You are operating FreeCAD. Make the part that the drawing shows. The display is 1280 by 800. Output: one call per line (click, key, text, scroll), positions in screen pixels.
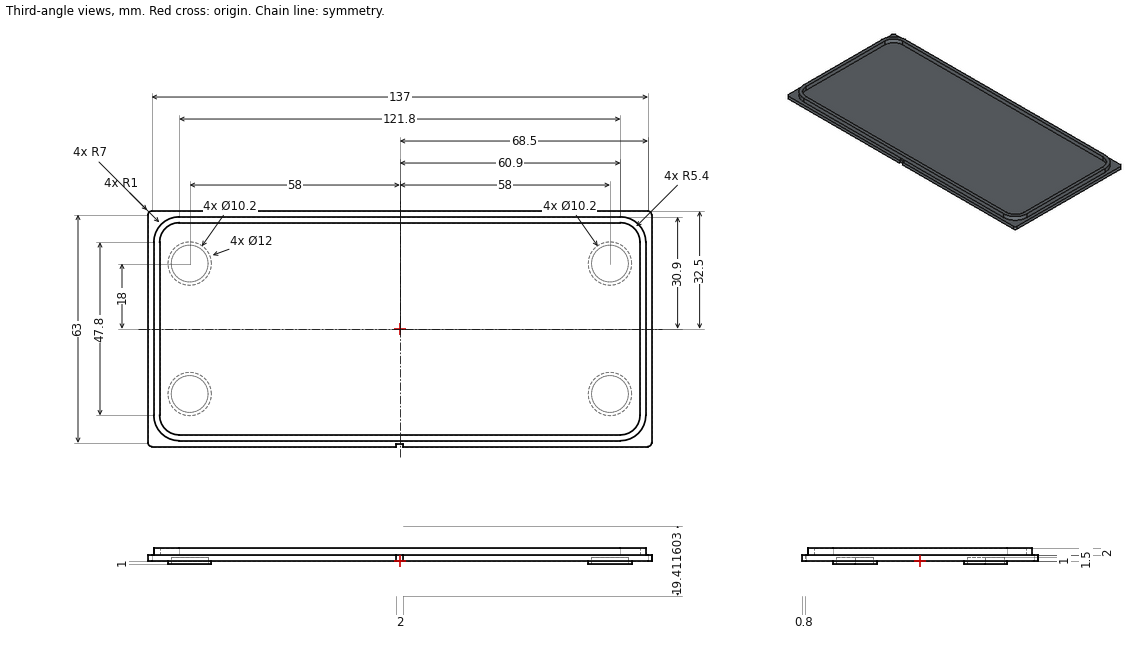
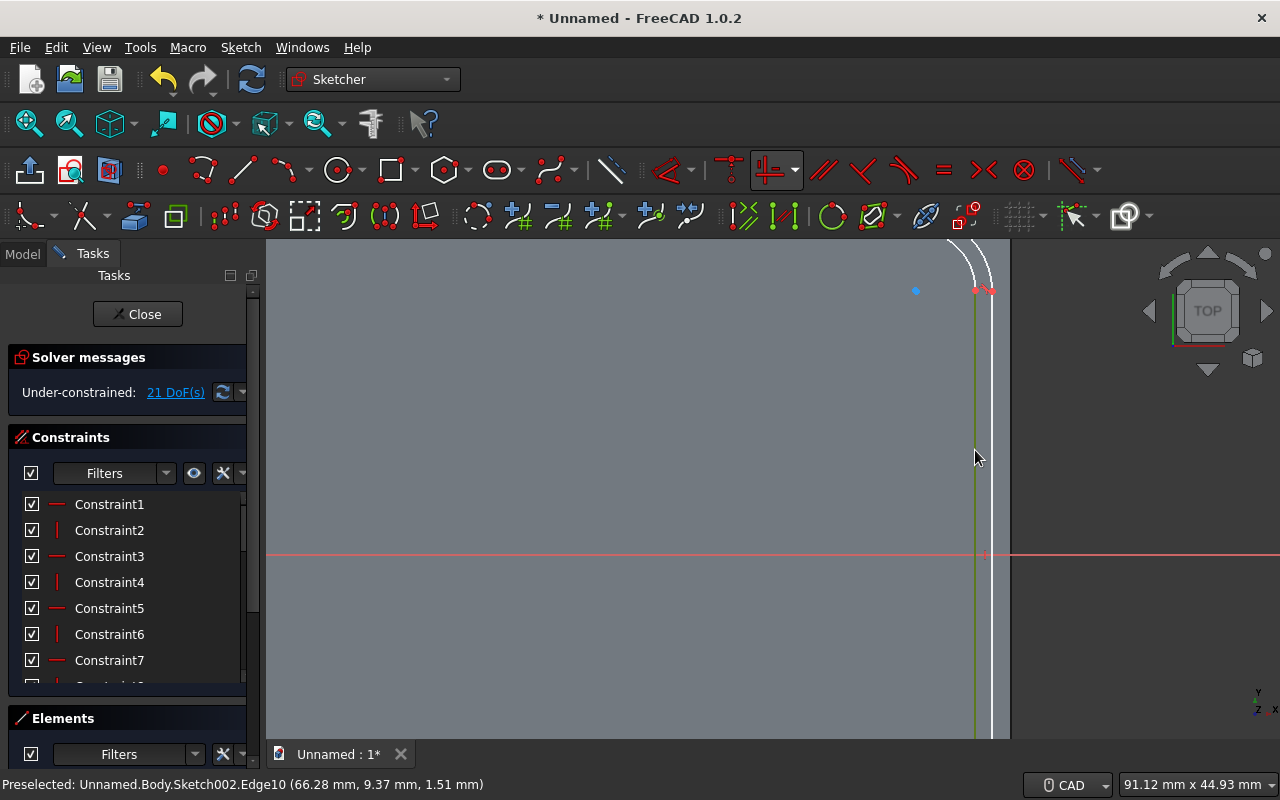
scroll(976, 450, down, 5)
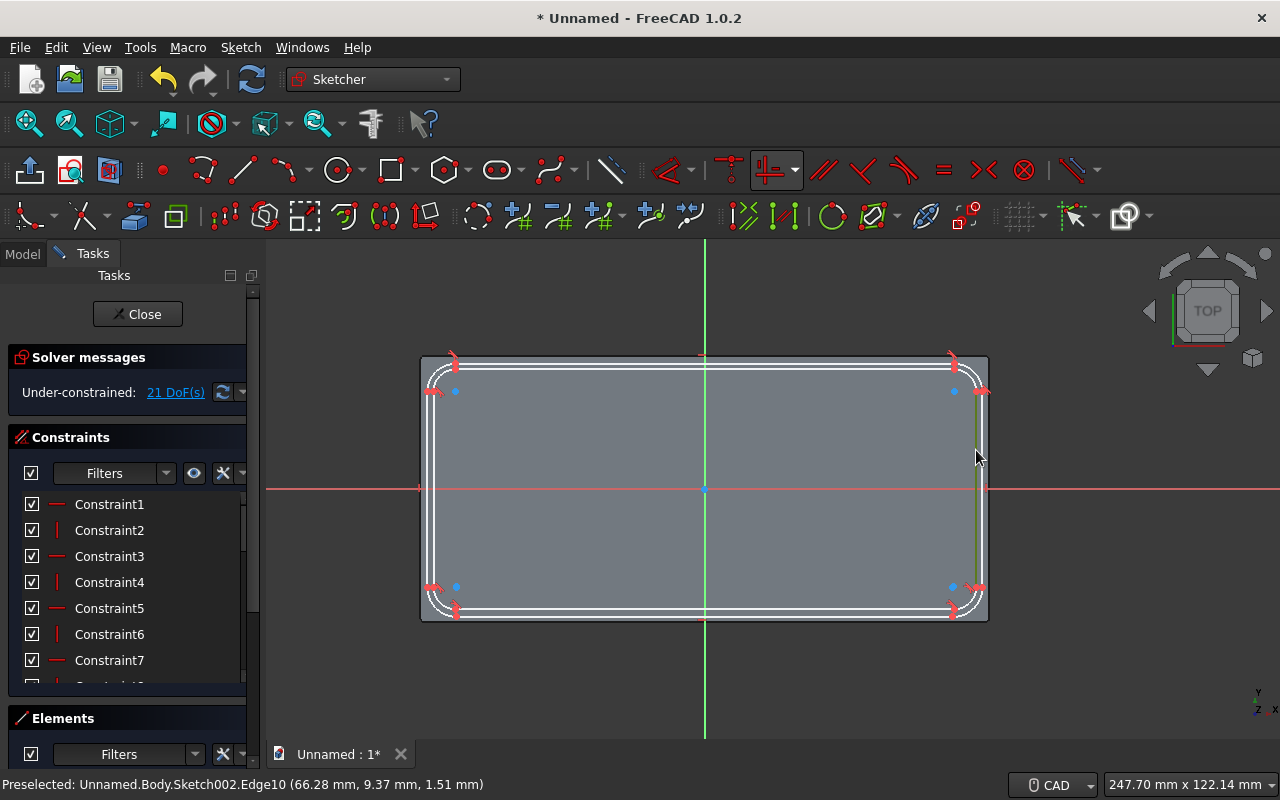
scroll(964, 607, up, 4)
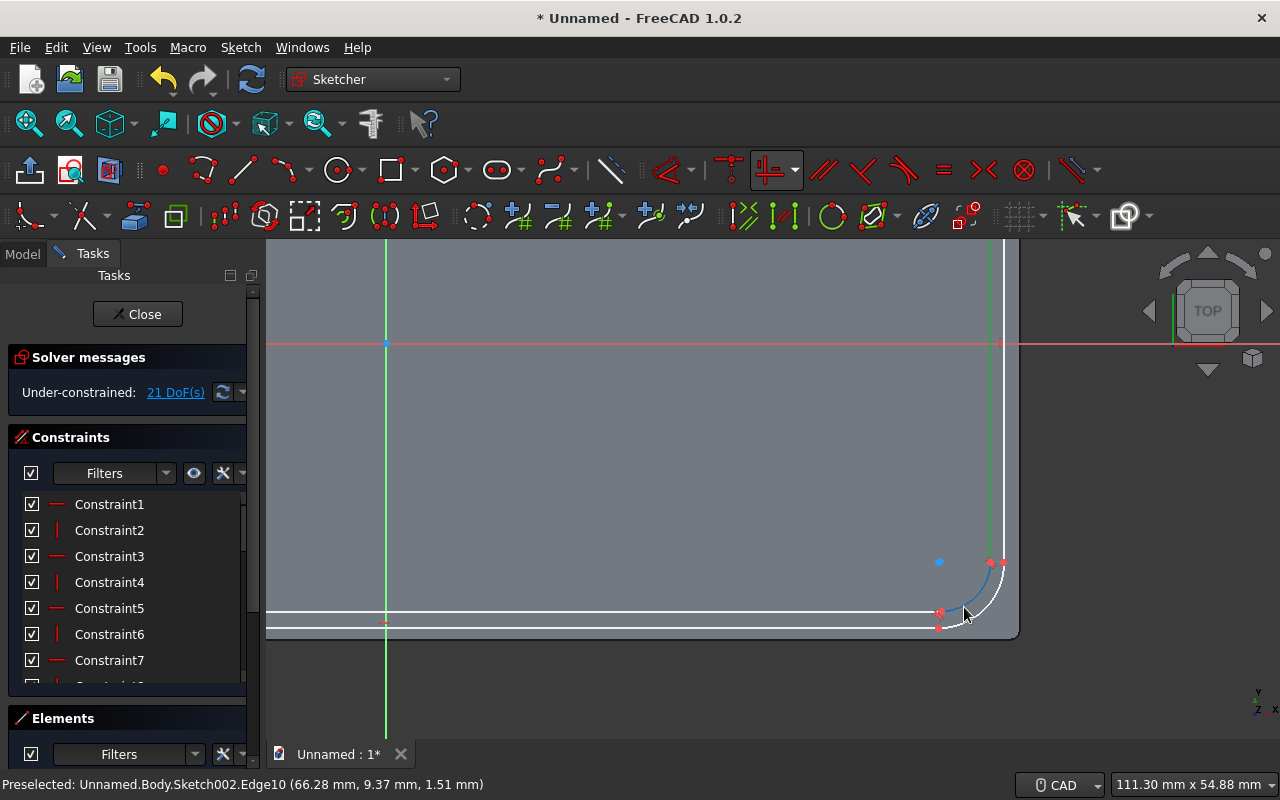
click(963, 606)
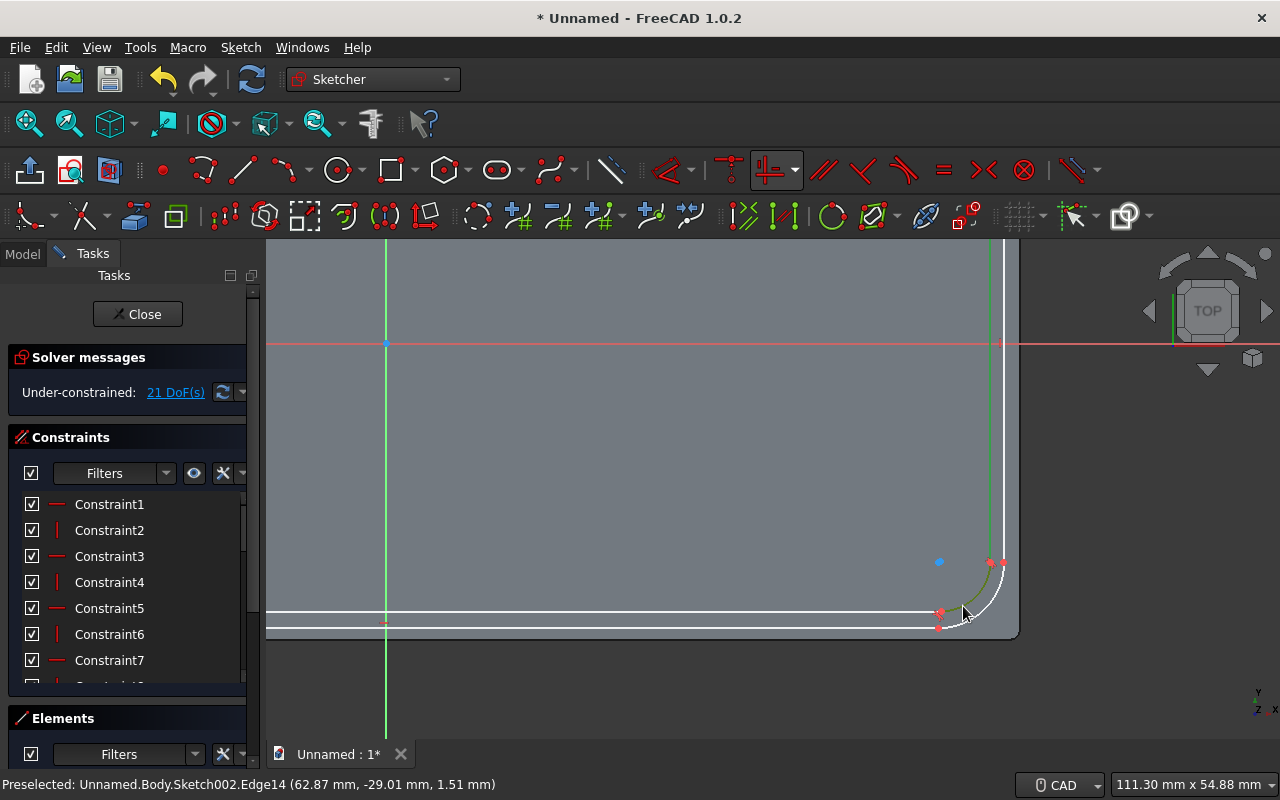
click(904, 170)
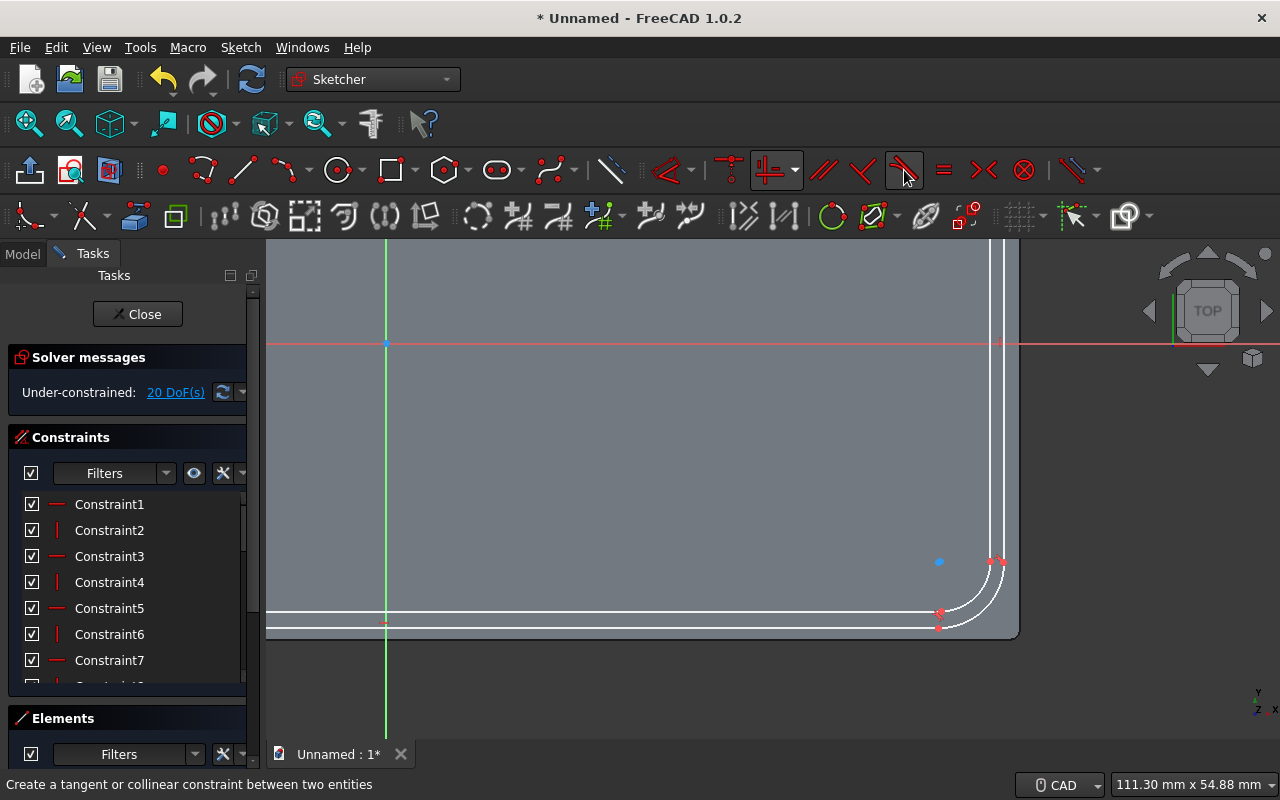
click(608, 612)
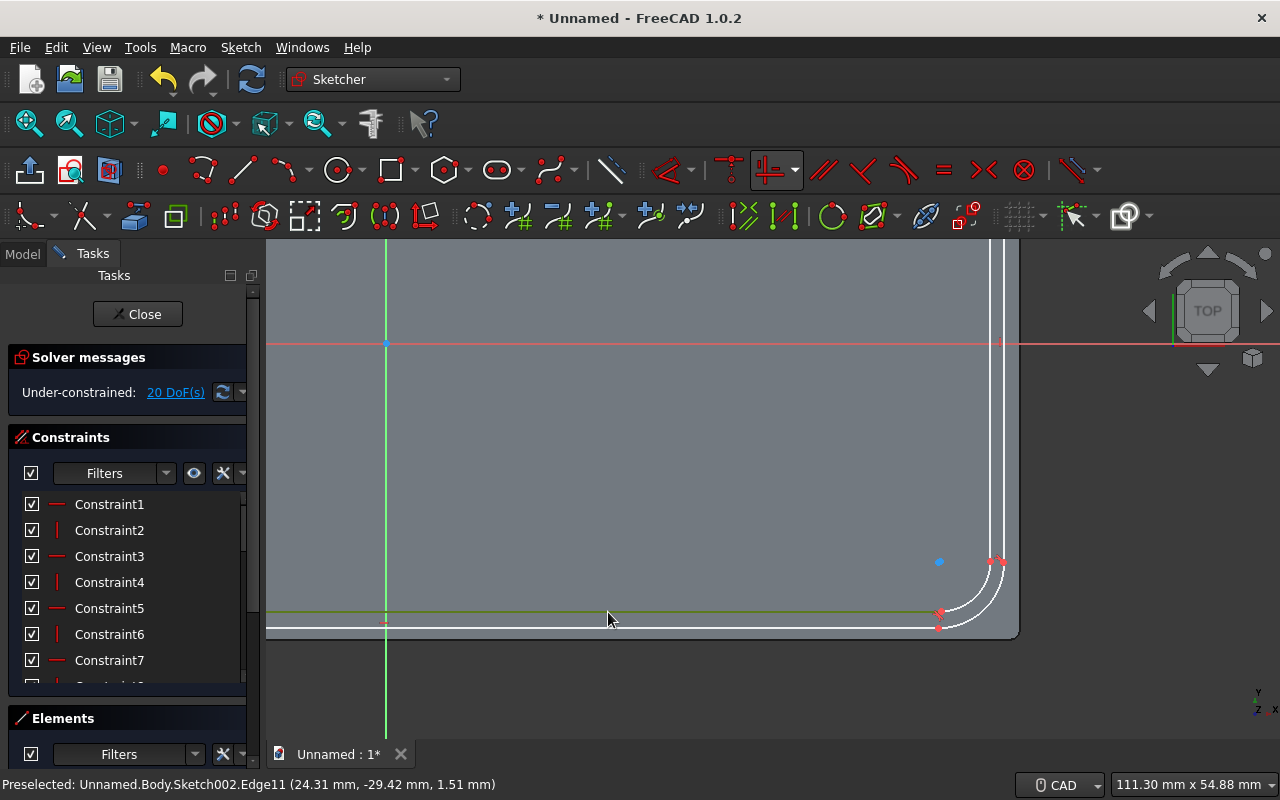
click(964, 606)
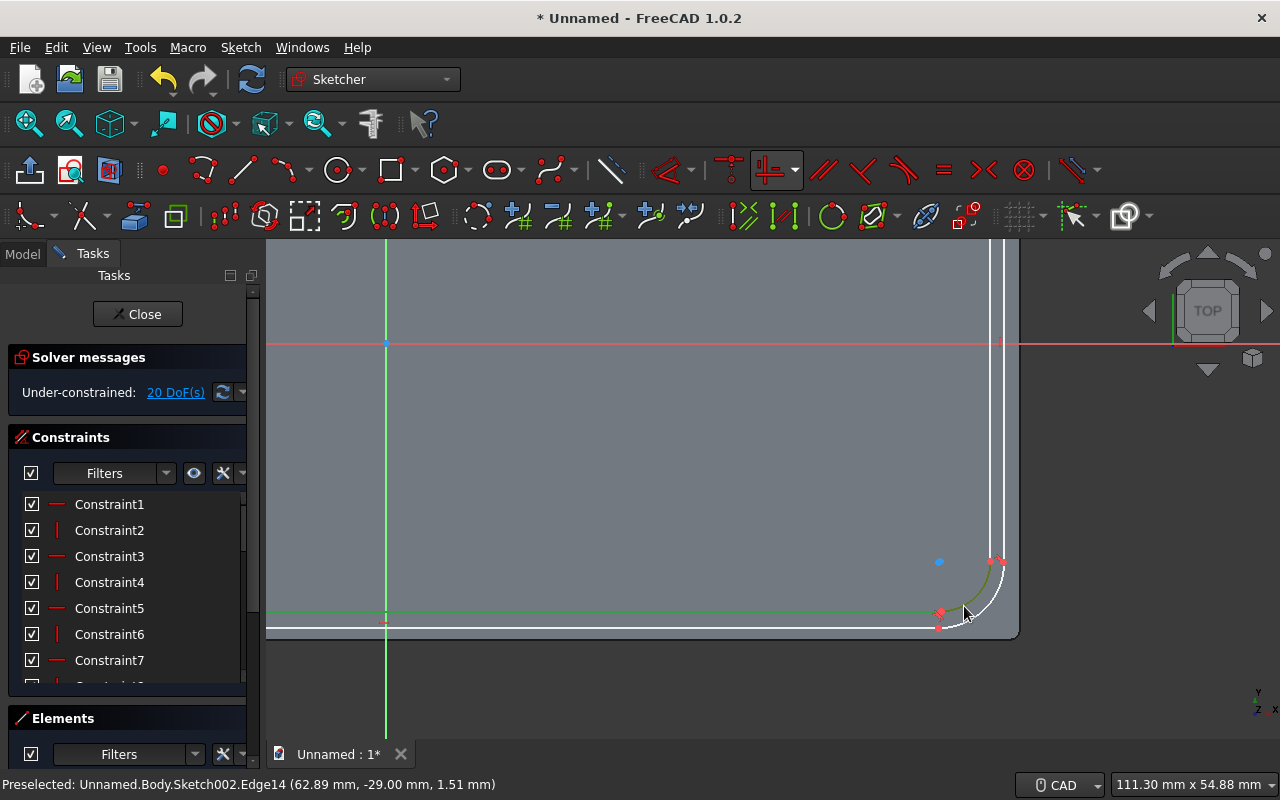
click(904, 170)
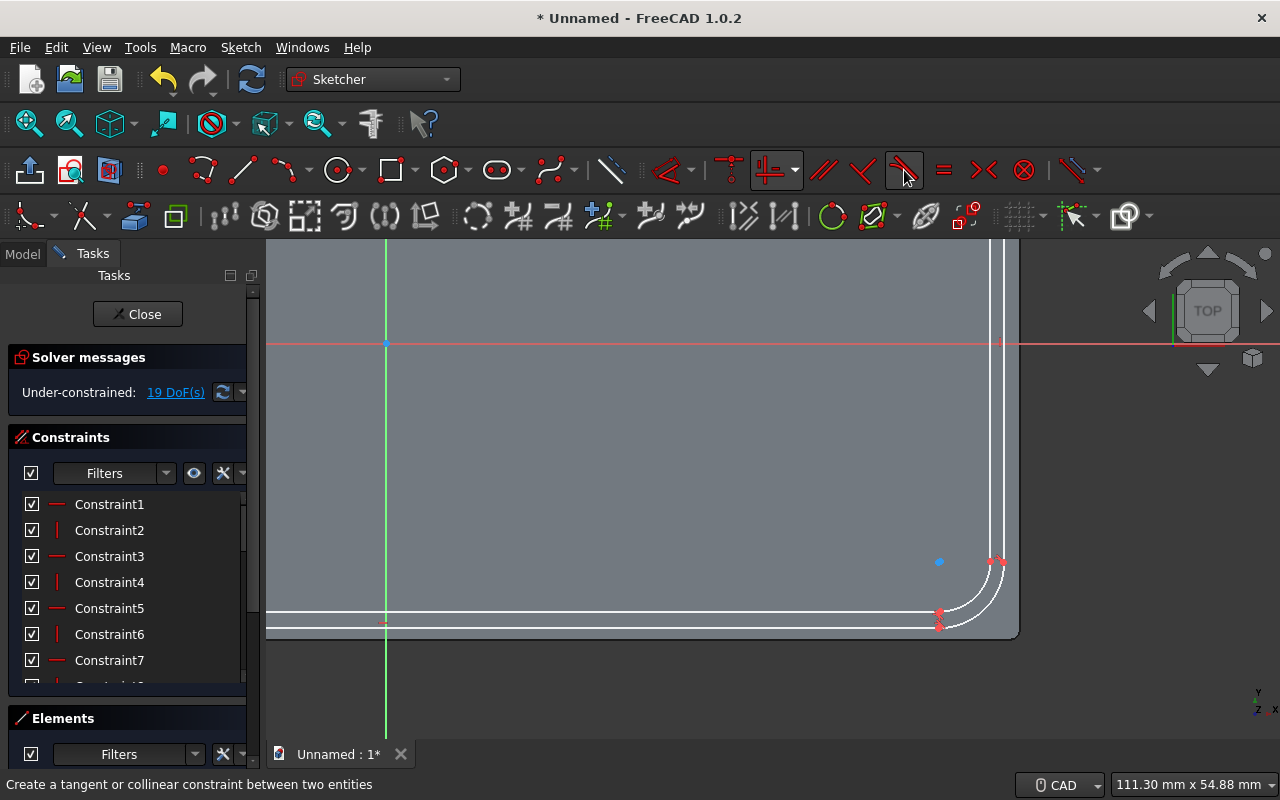
click(608, 612)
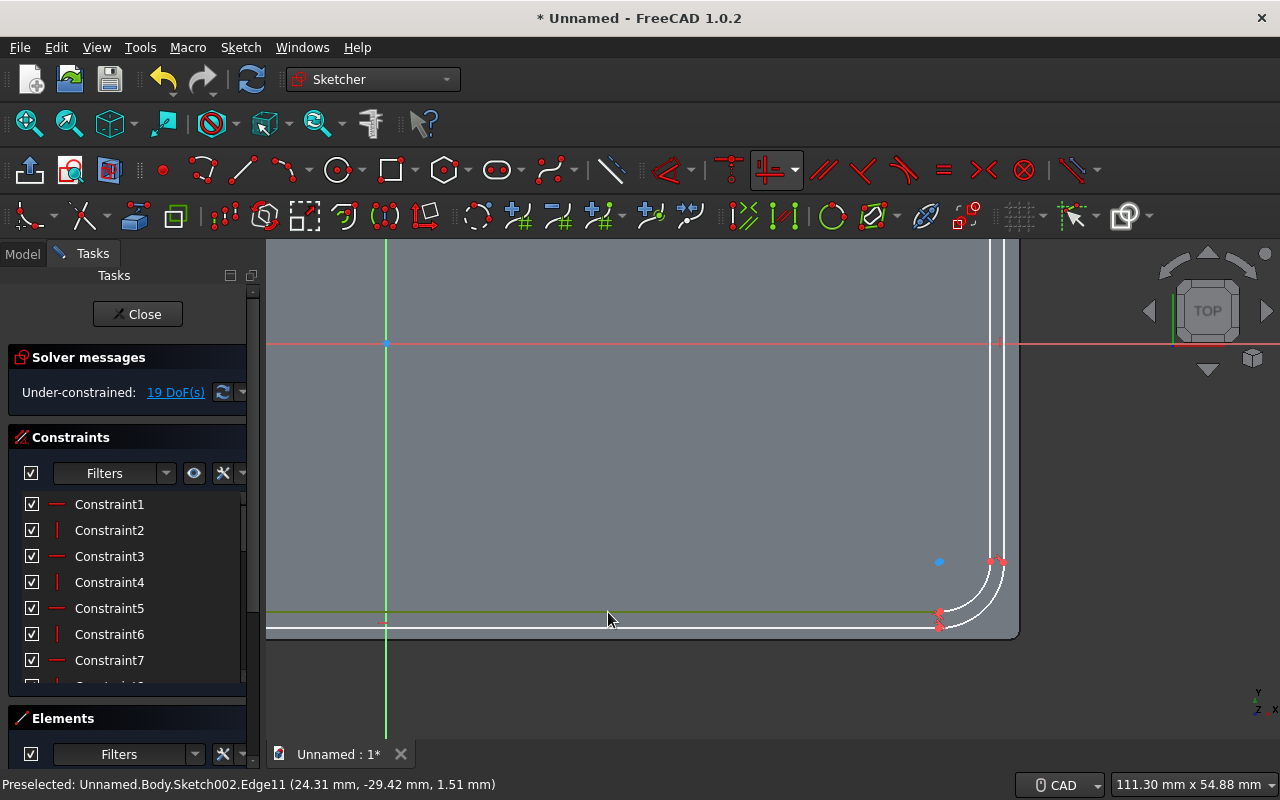
scroll(964, 608, down, 4)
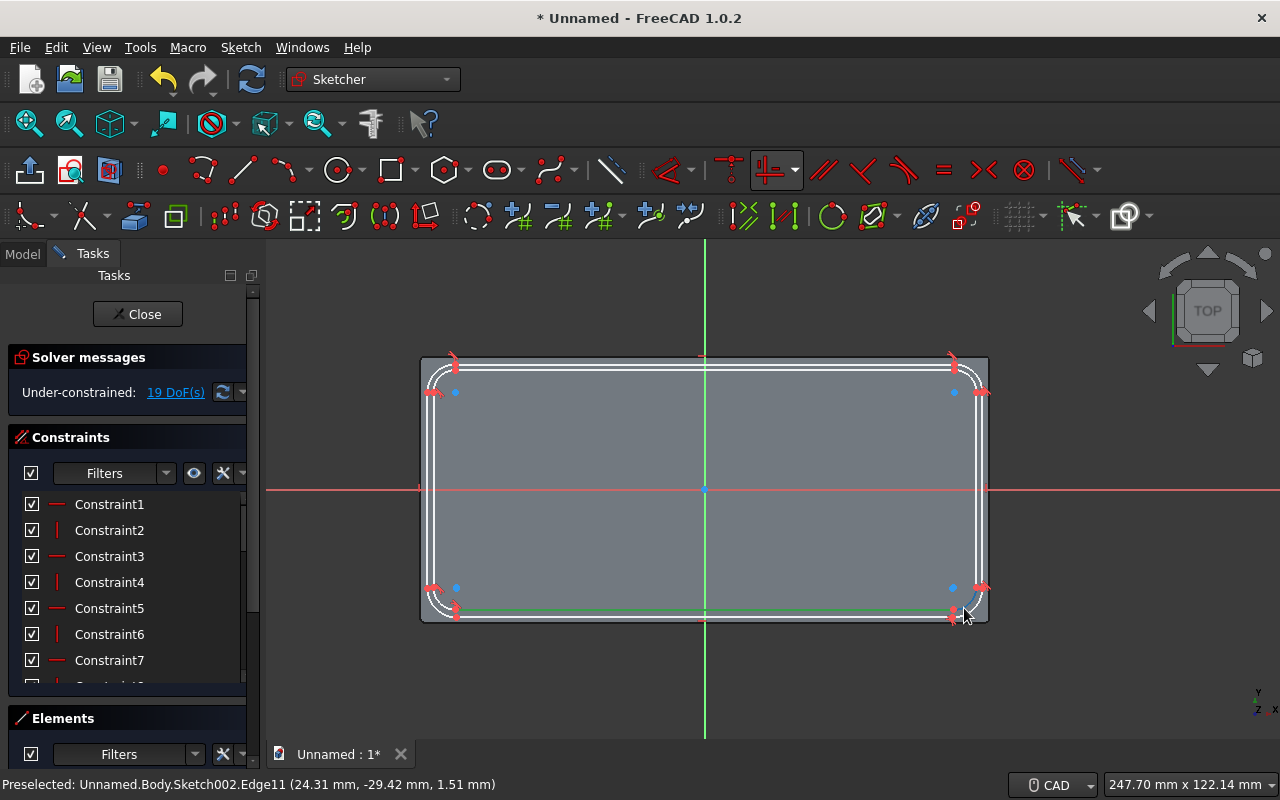
scroll(436, 598, up, 4)